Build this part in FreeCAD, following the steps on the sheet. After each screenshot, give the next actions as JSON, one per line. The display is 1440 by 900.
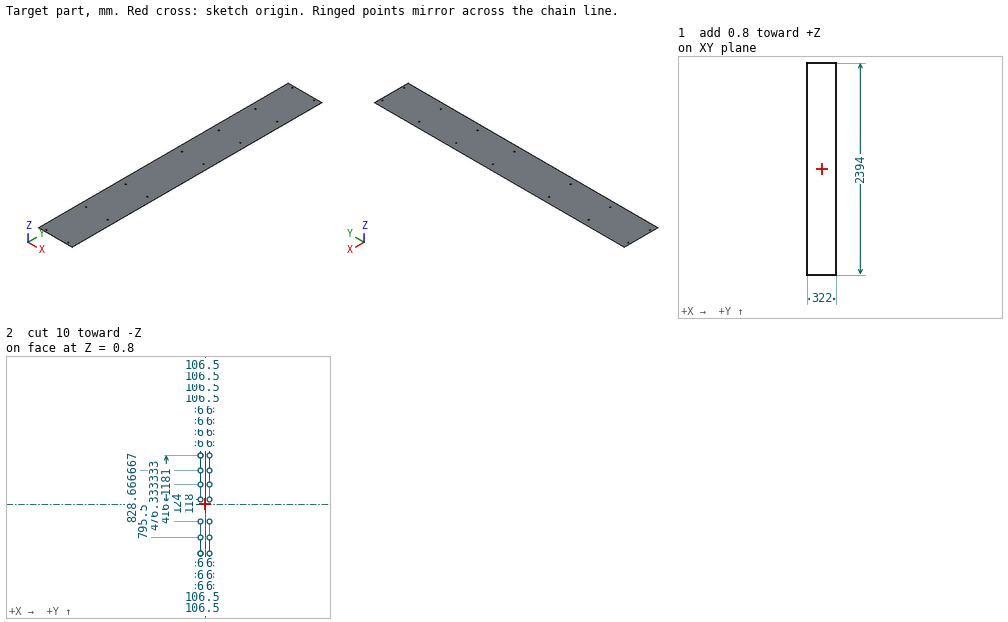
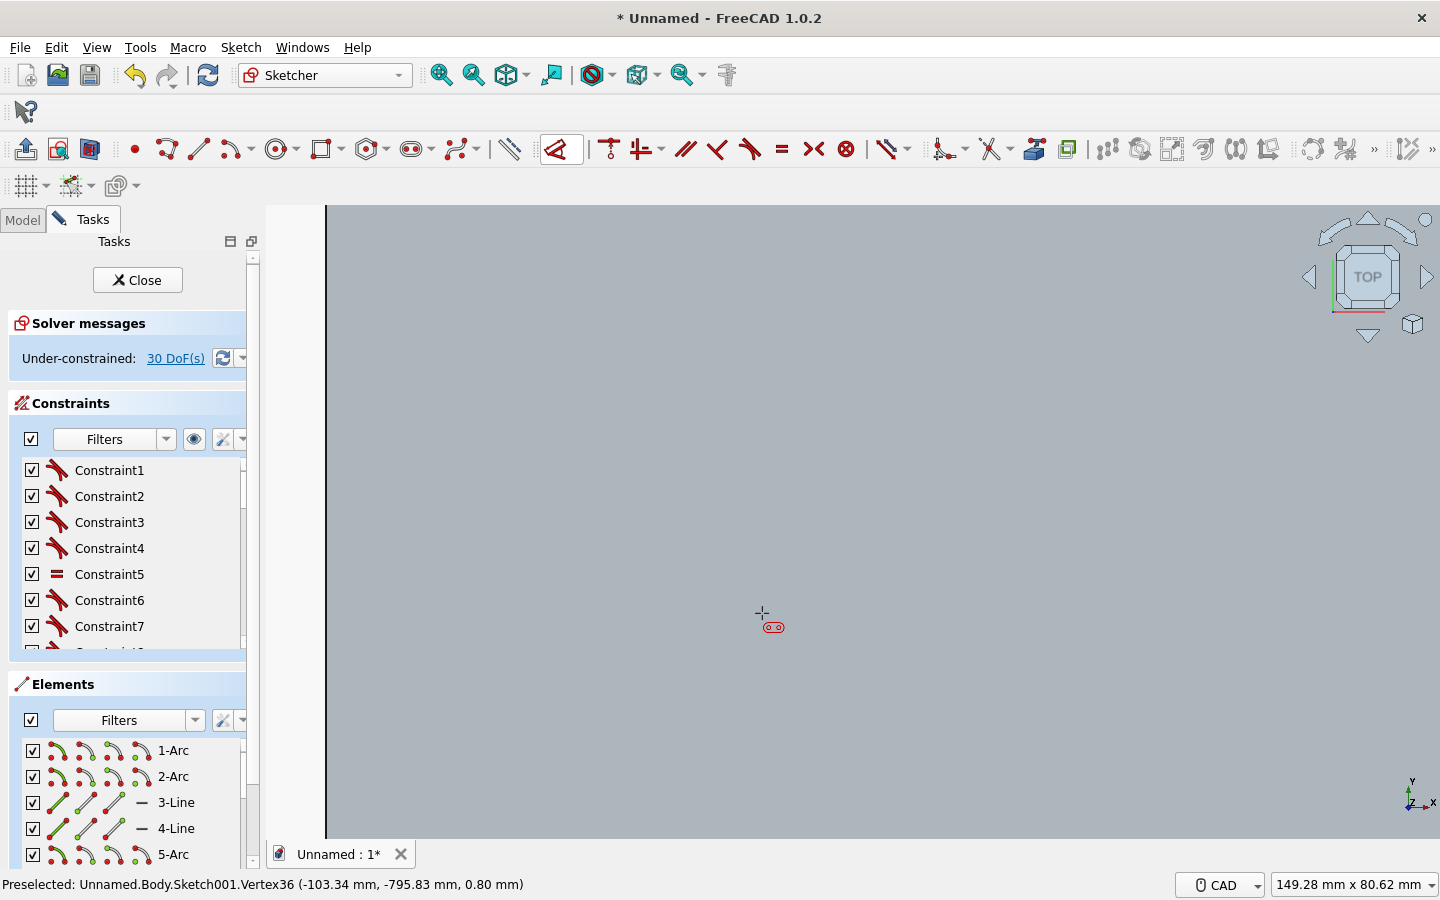
{"action": "scroll", "coordinate": [762, 613], "scroll_direction": "down", "scroll_amount": 18}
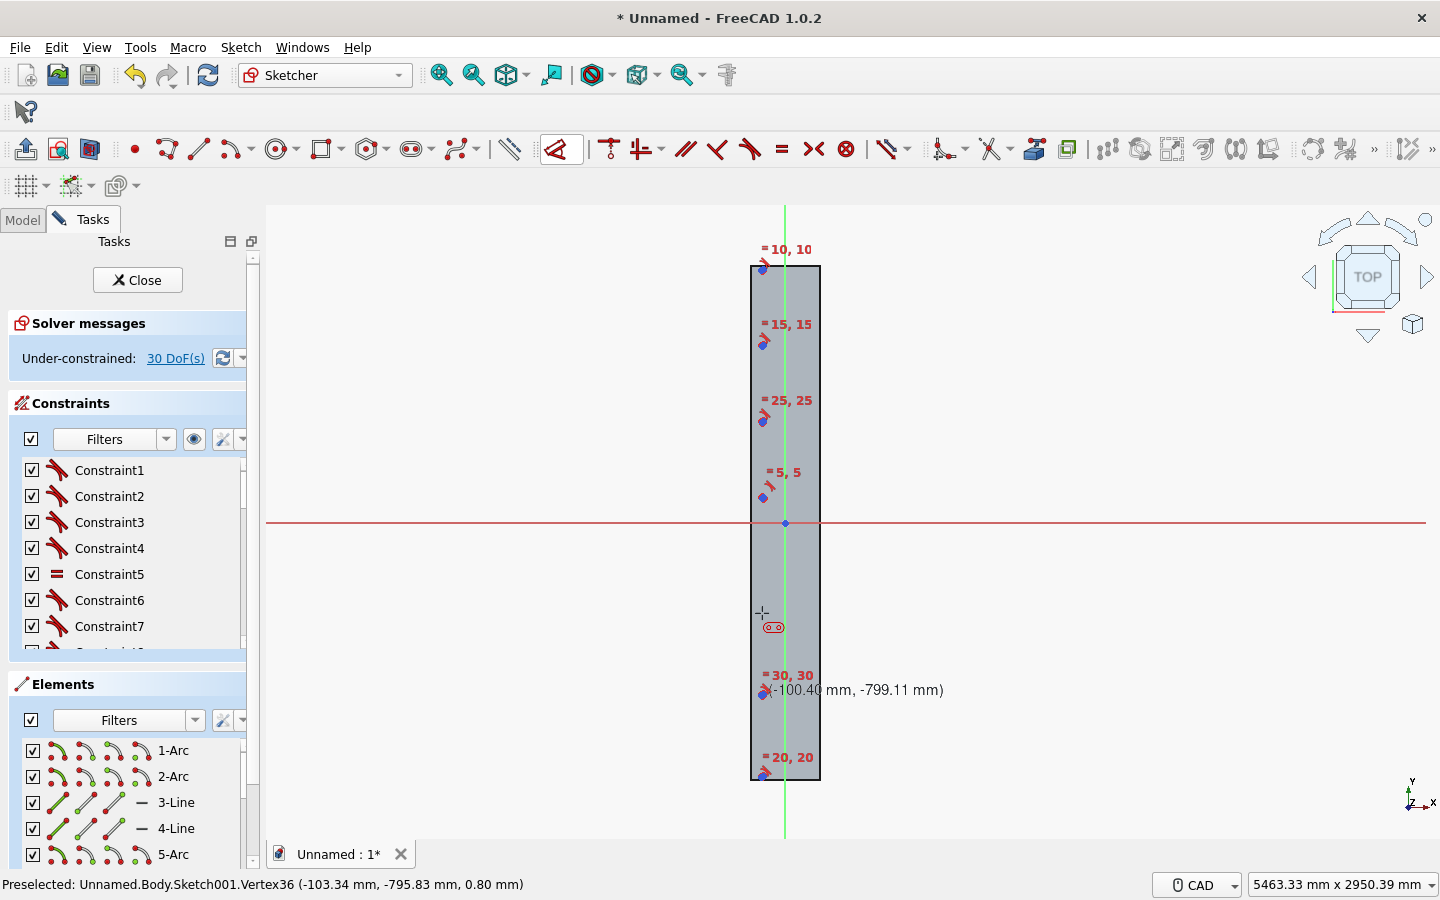
{"action": "left_click", "coordinate": [762, 613]}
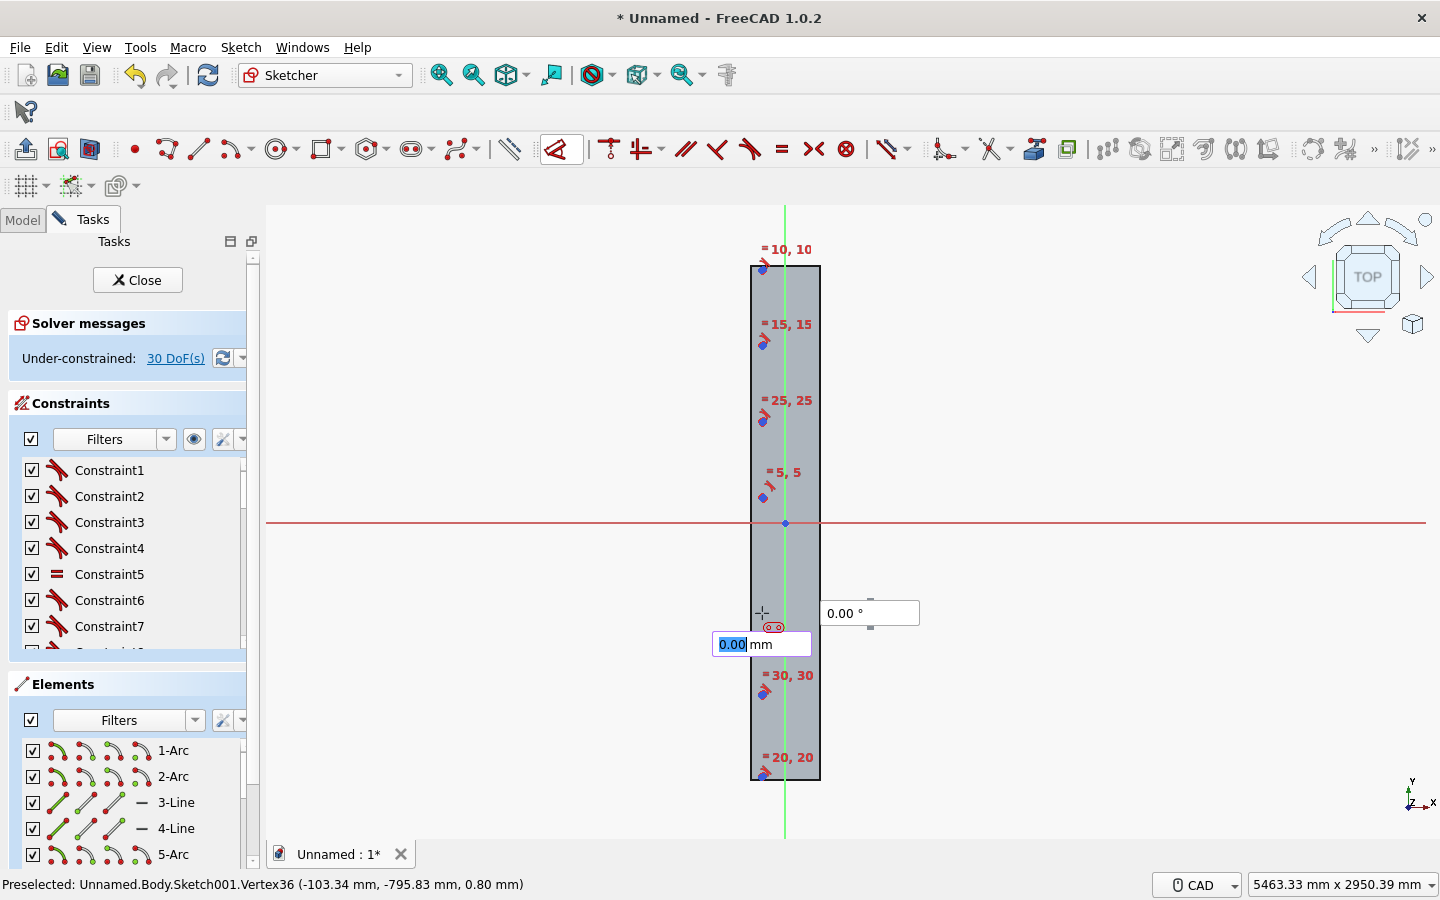
{"action": "scroll", "coordinate": [764, 613], "scroll_direction": "up", "scroll_amount": 13}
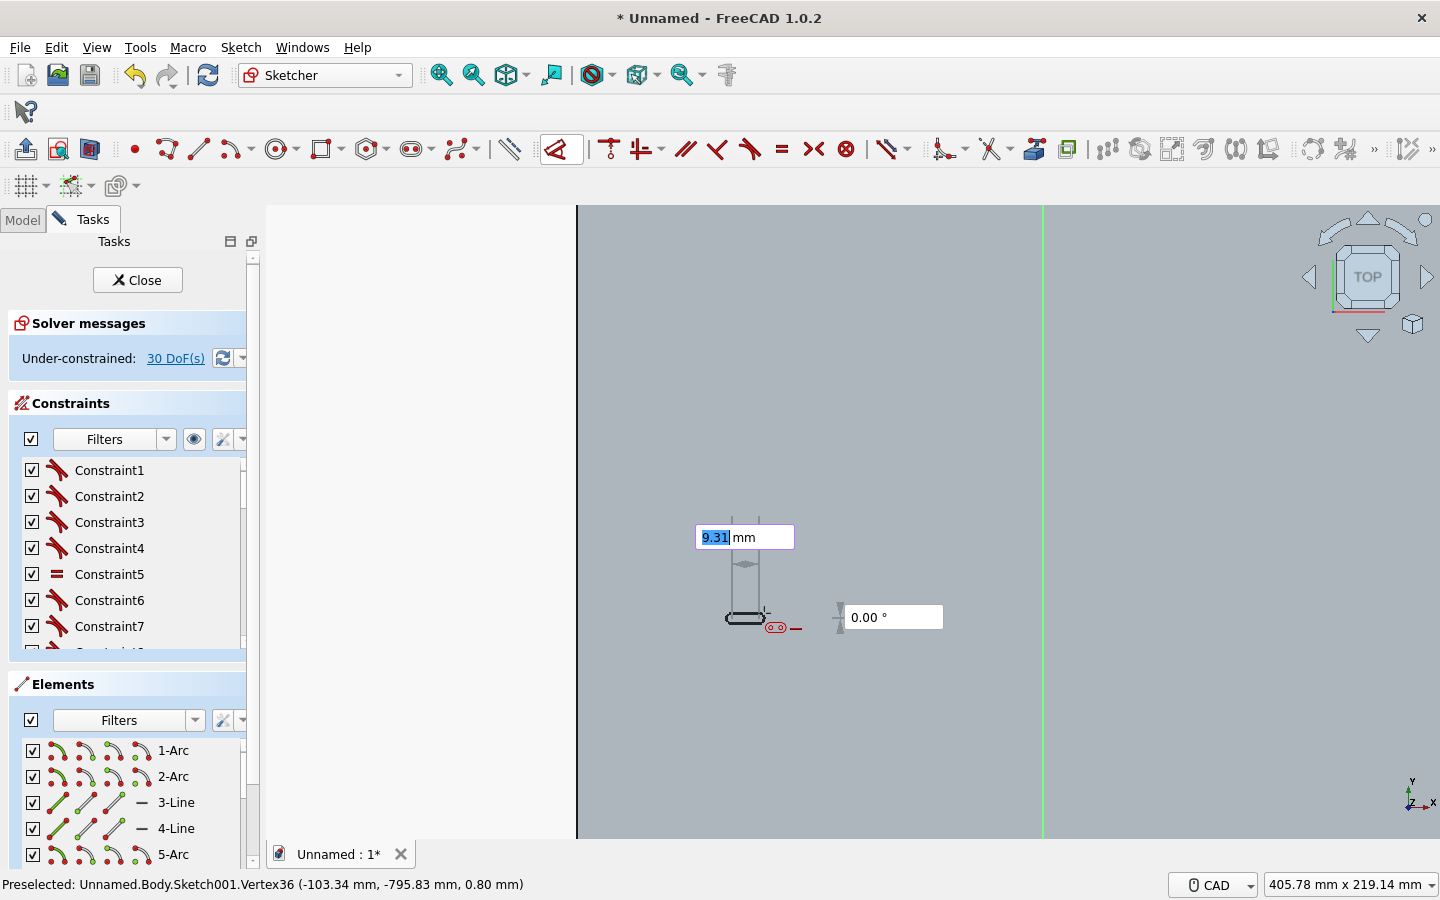
{"action": "left_click", "coordinate": [752, 605]}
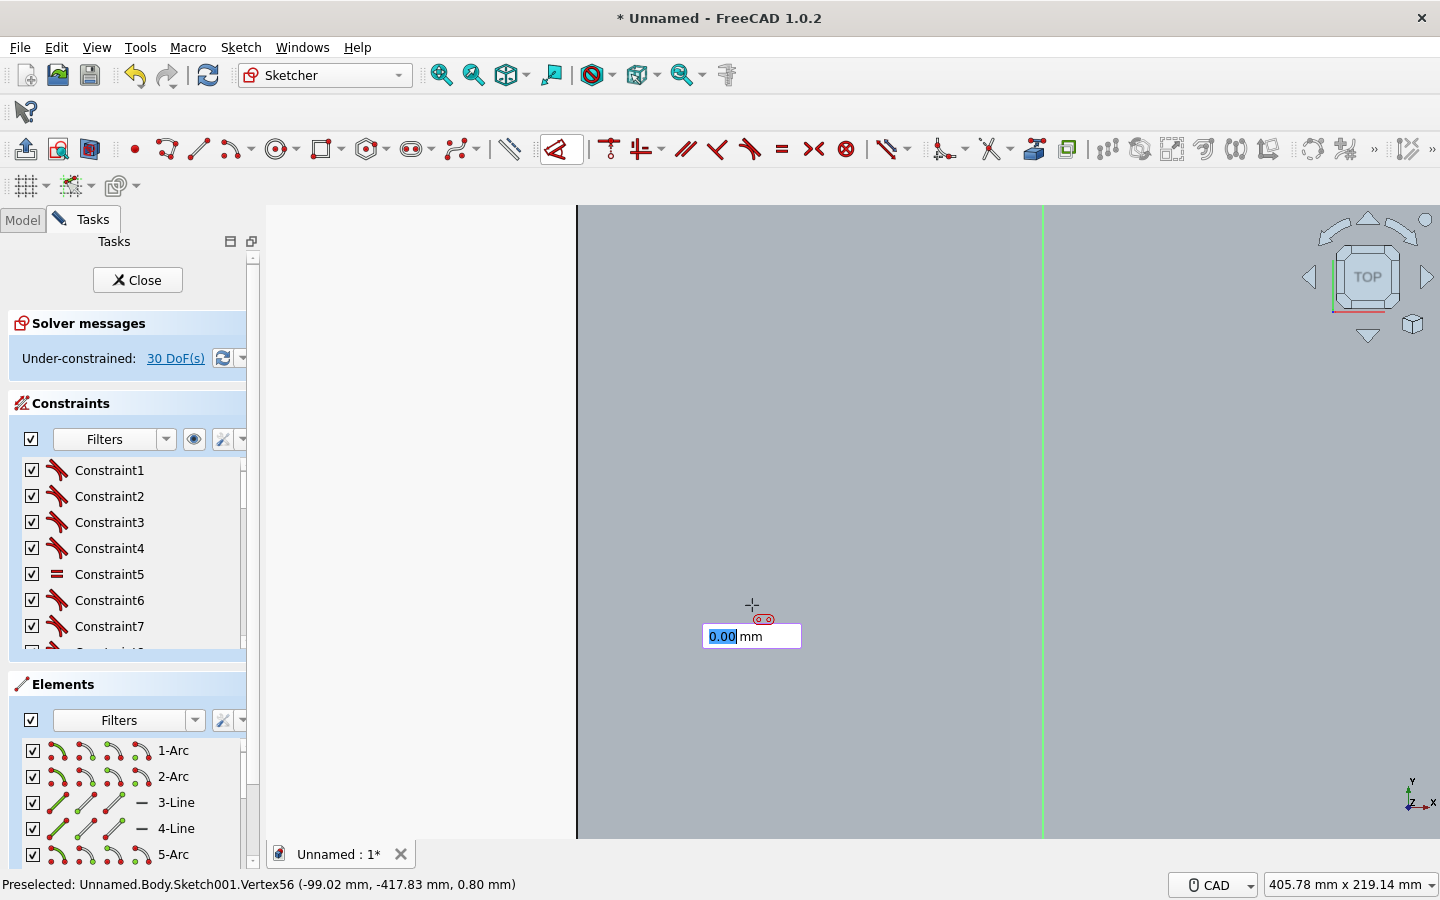
{"action": "scroll", "coordinate": [743, 598], "scroll_direction": "up", "scroll_amount": 4}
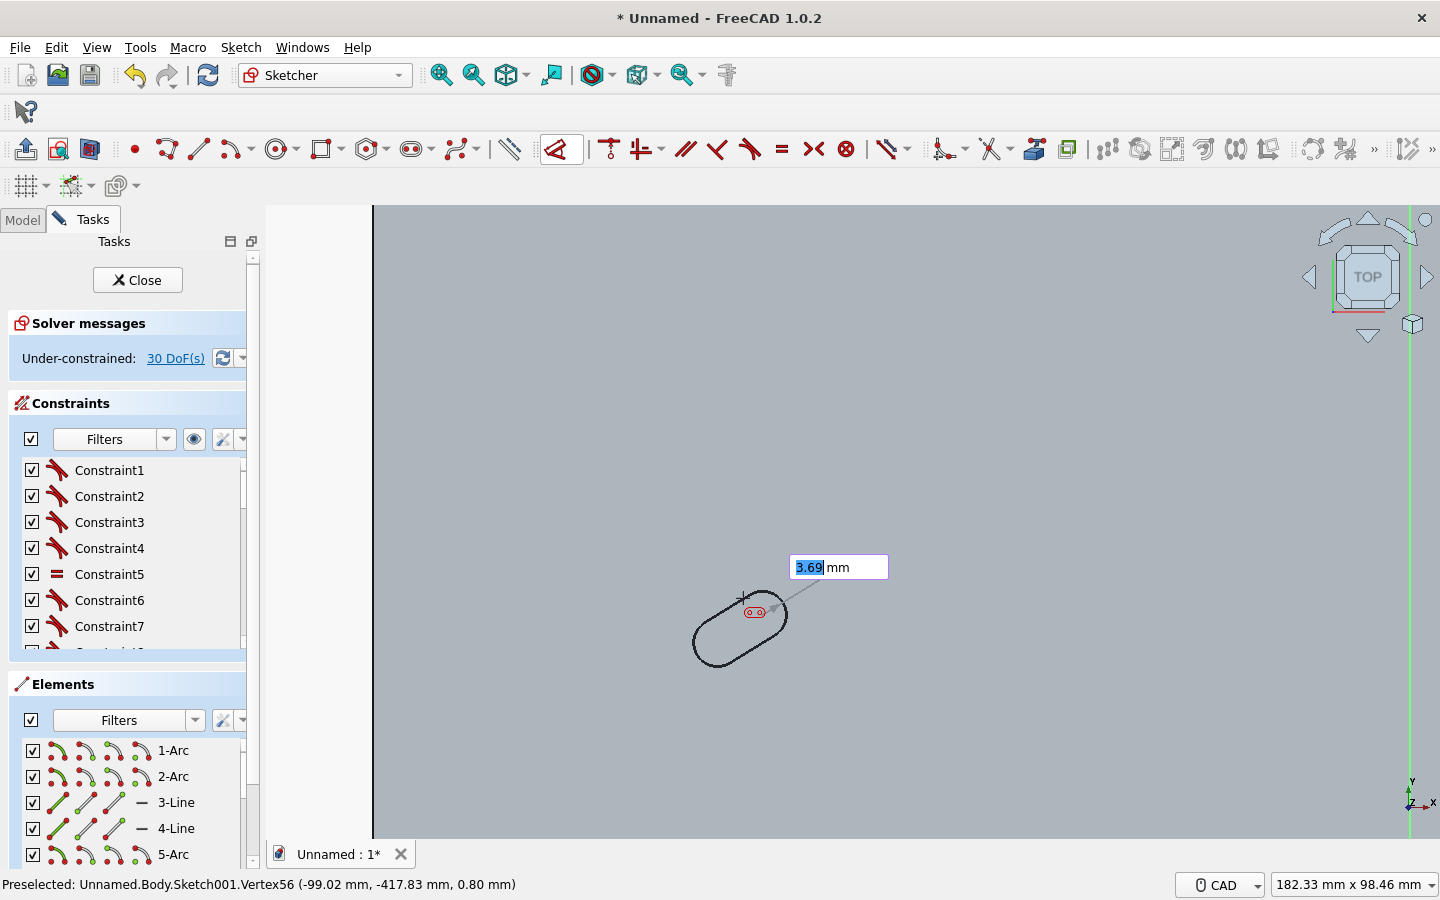
{"action": "left_click", "coordinate": [743, 598]}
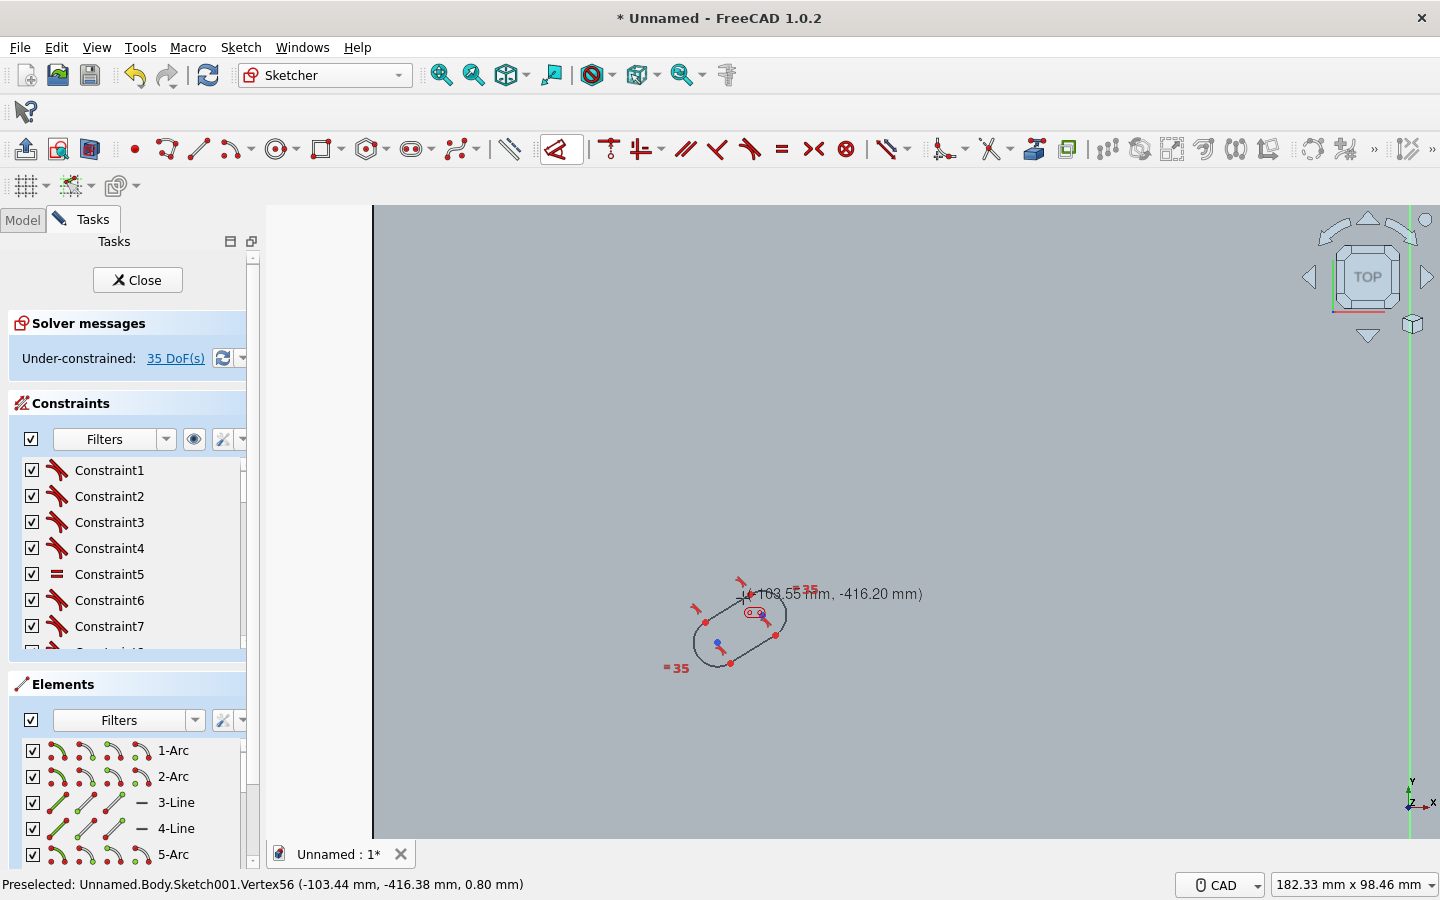
{"action": "scroll", "coordinate": [763, 612], "scroll_direction": "down", "scroll_amount": 17}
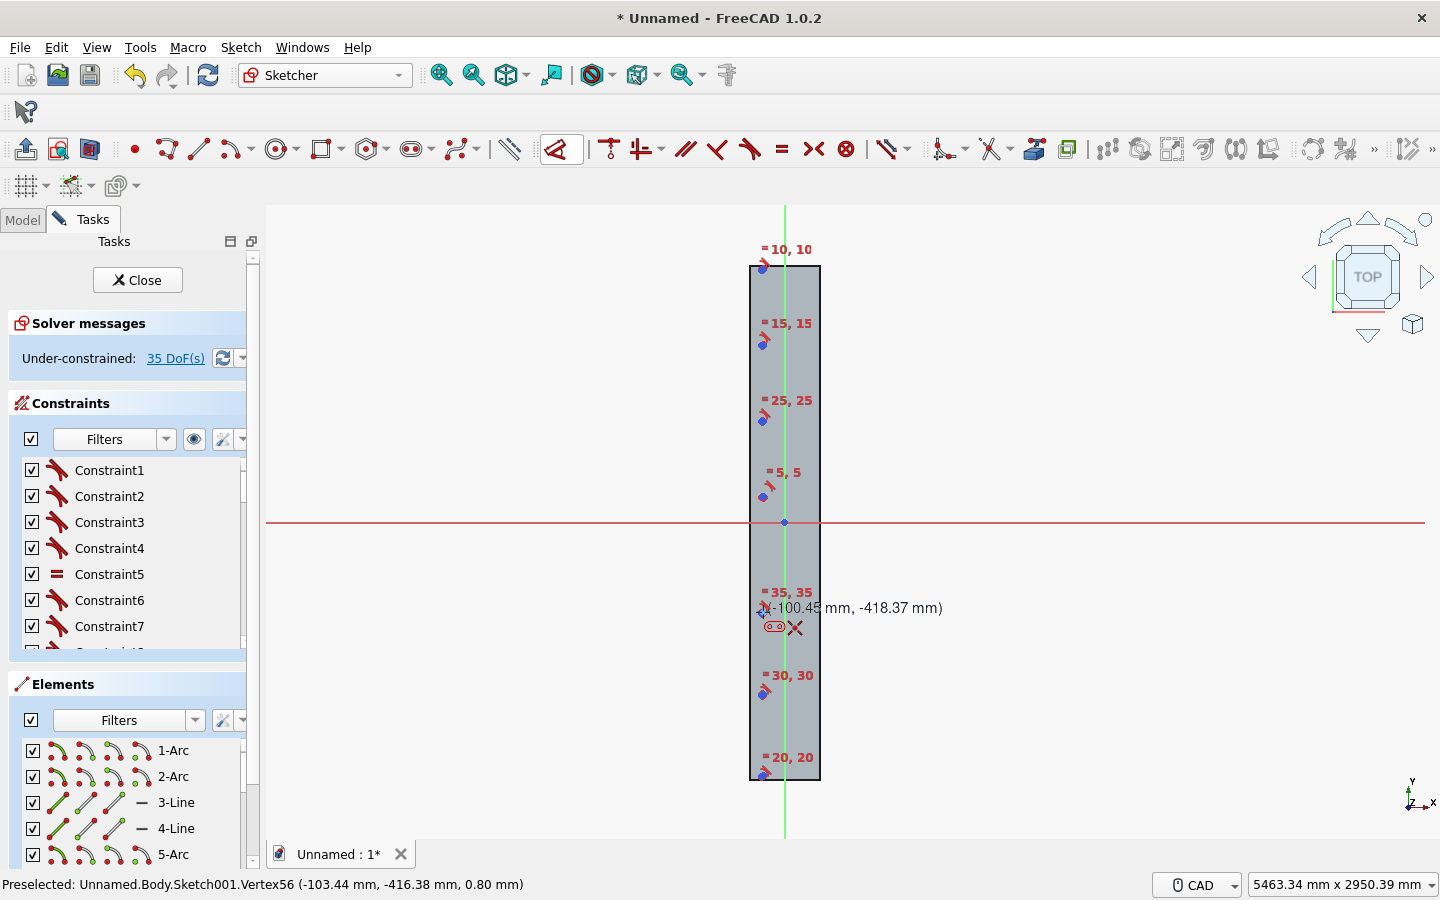
{"action": "scroll", "coordinate": [807, 776], "scroll_direction": "up", "scroll_amount": 18}